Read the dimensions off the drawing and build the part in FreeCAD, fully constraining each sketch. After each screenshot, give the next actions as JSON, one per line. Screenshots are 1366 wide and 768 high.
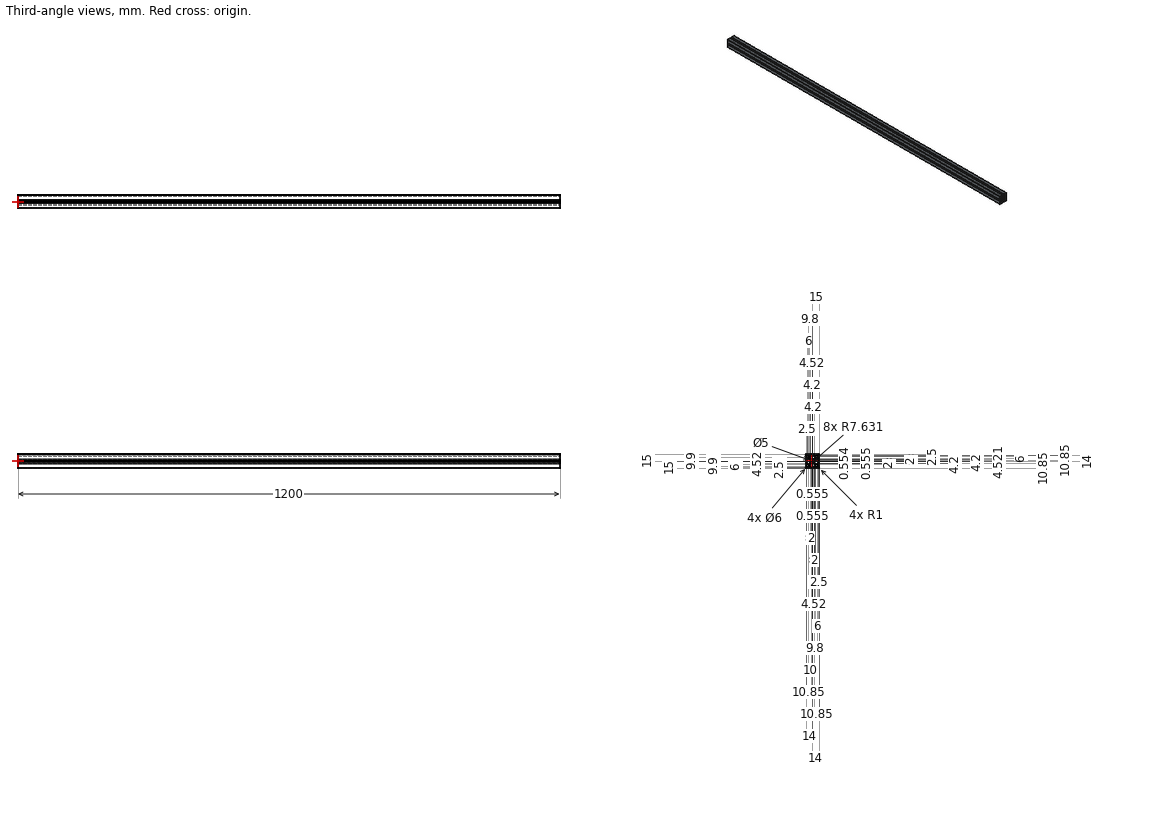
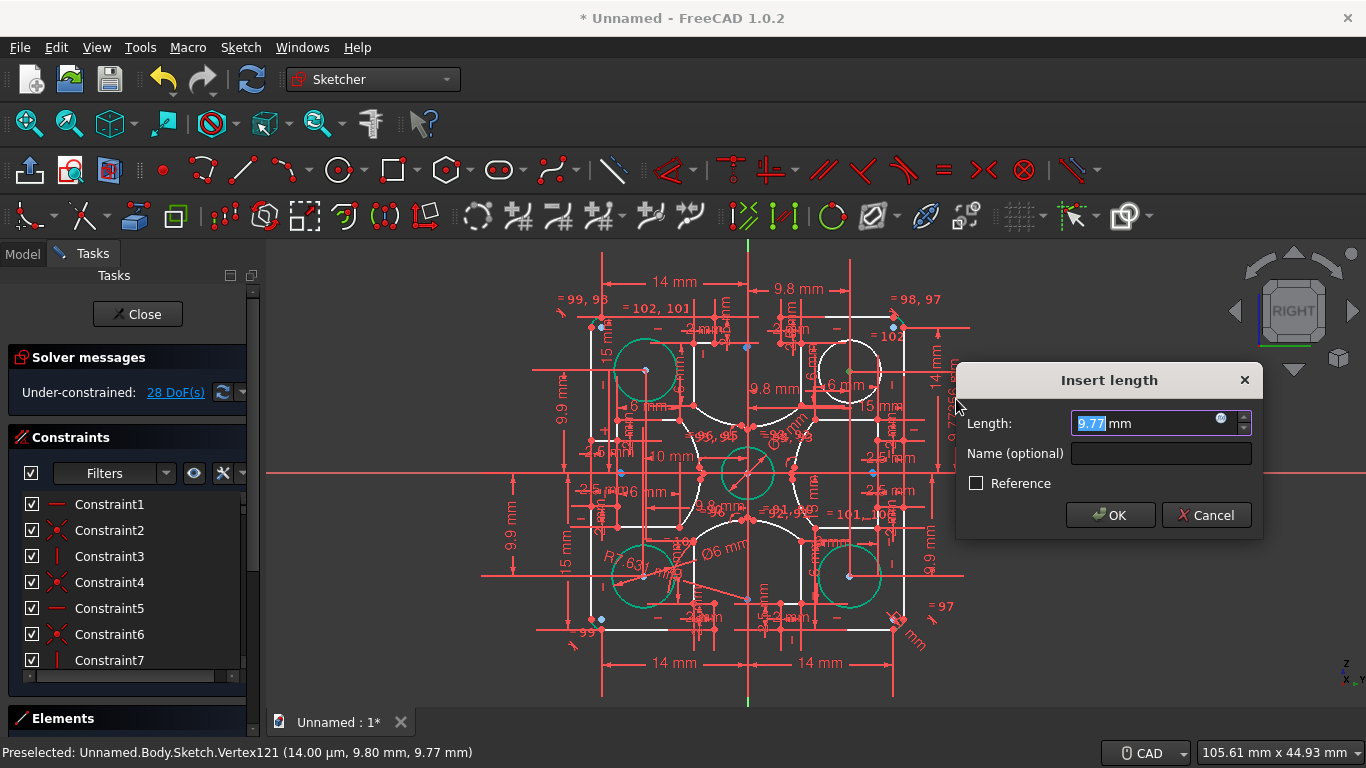
{"action": "type", "text": "9.9"}
{"action": "key", "text": "Return"}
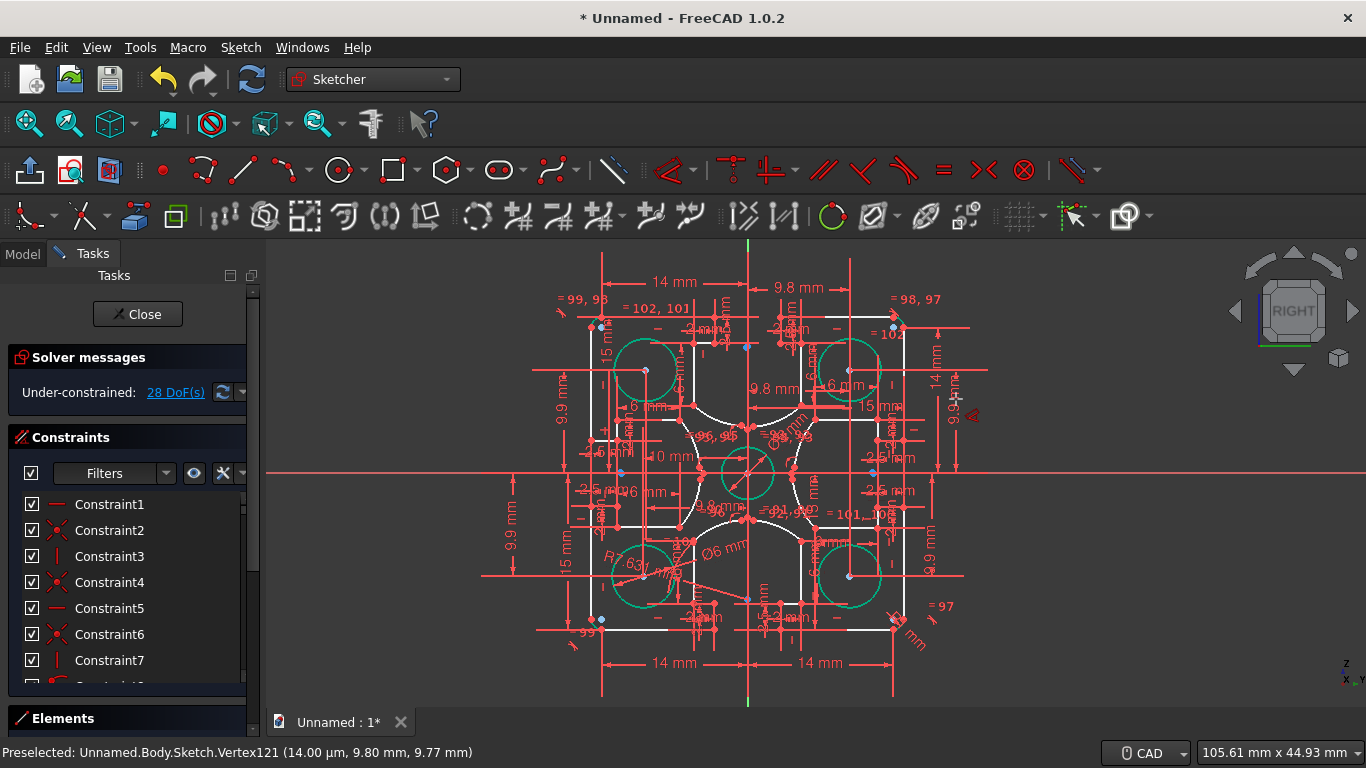
{"action": "scroll", "coordinate": [748, 517], "scroll_direction": "up", "scroll_amount": 4}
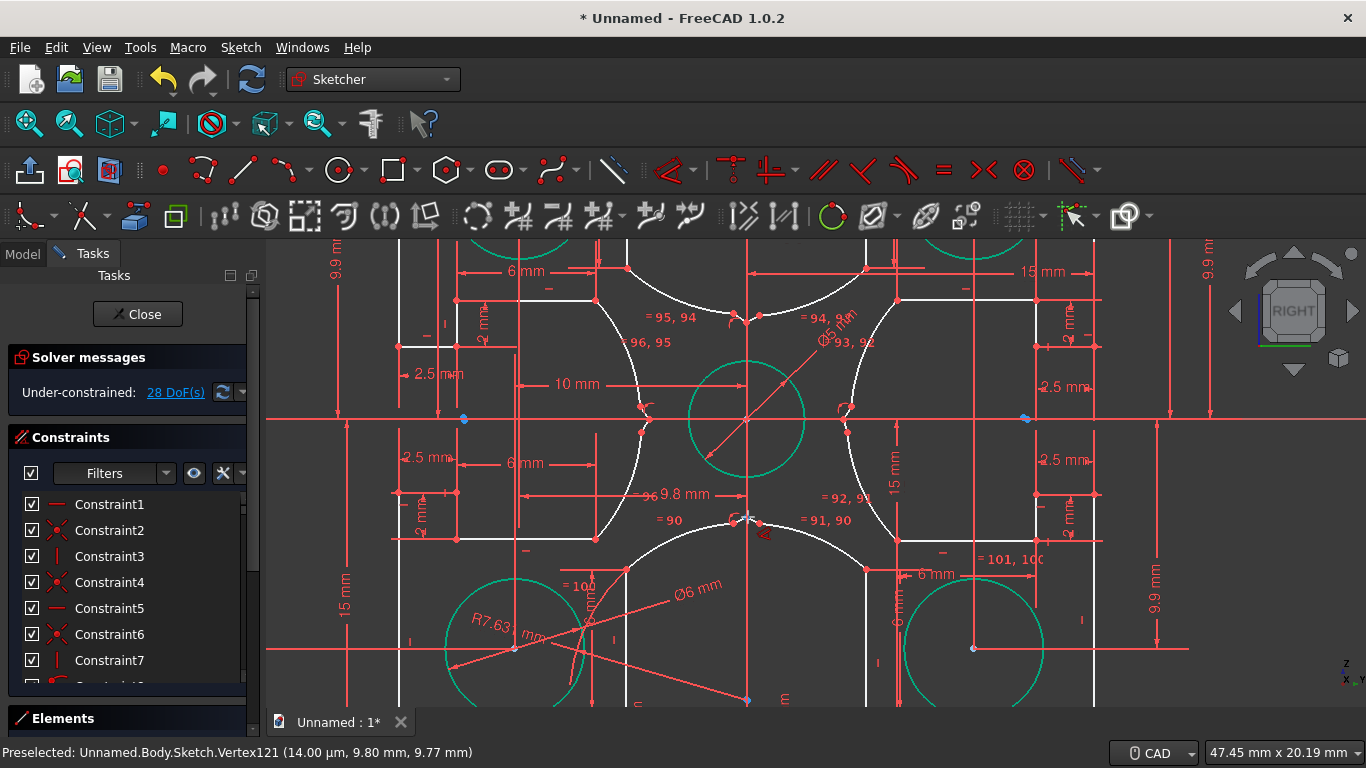
{"action": "left_click", "coordinate": [747, 517]}
{"action": "left_click", "coordinate": [781, 446]}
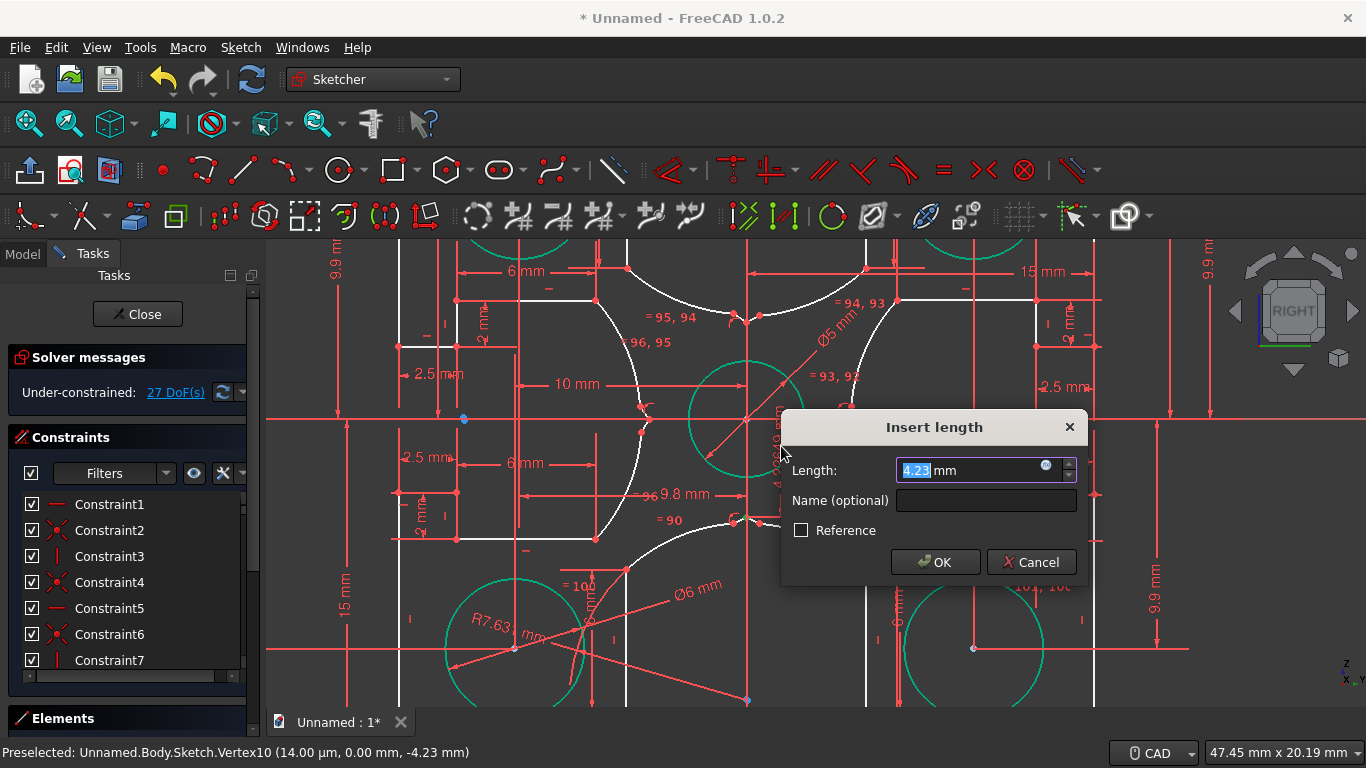
{"action": "type", "text": "4.2"}
{"action": "key", "text": "Return"}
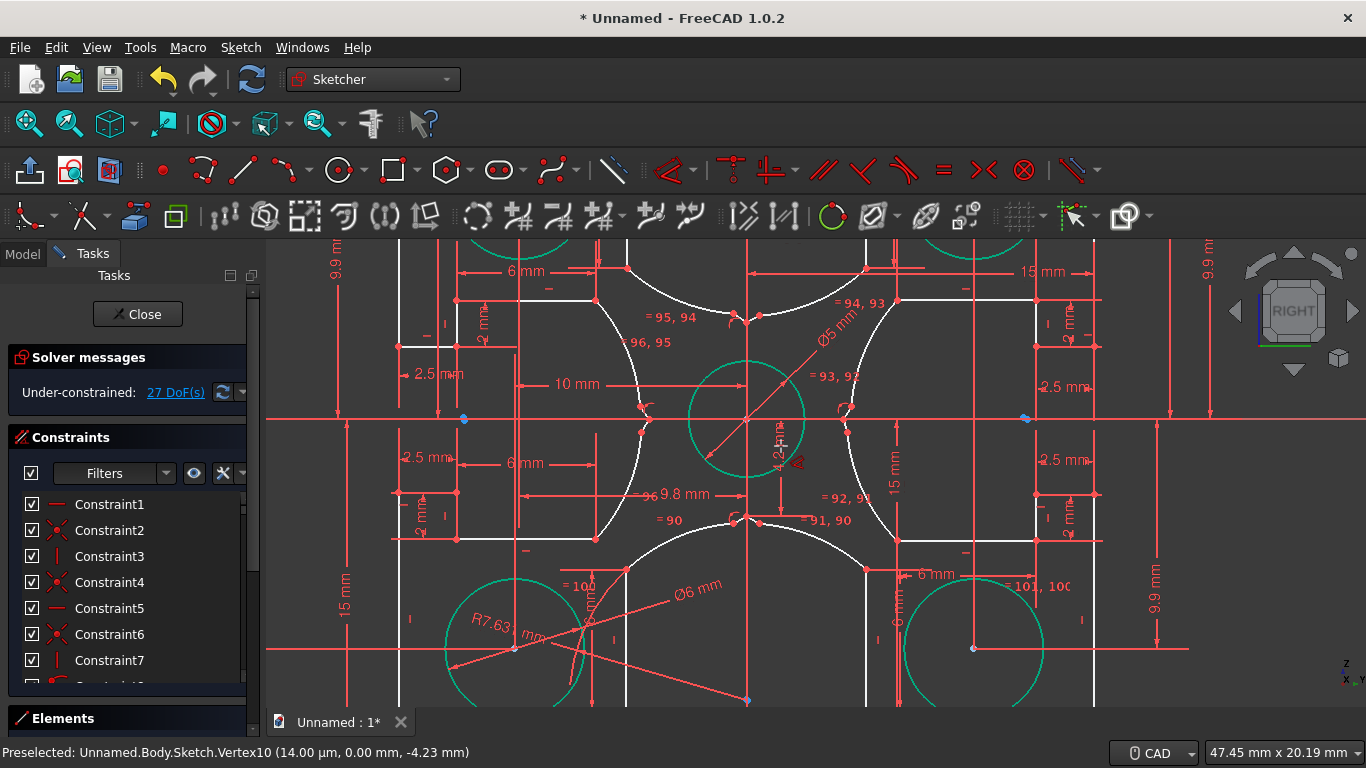
{"action": "left_click", "coordinate": [844, 419]}
{"action": "left_click", "coordinate": [773, 385]}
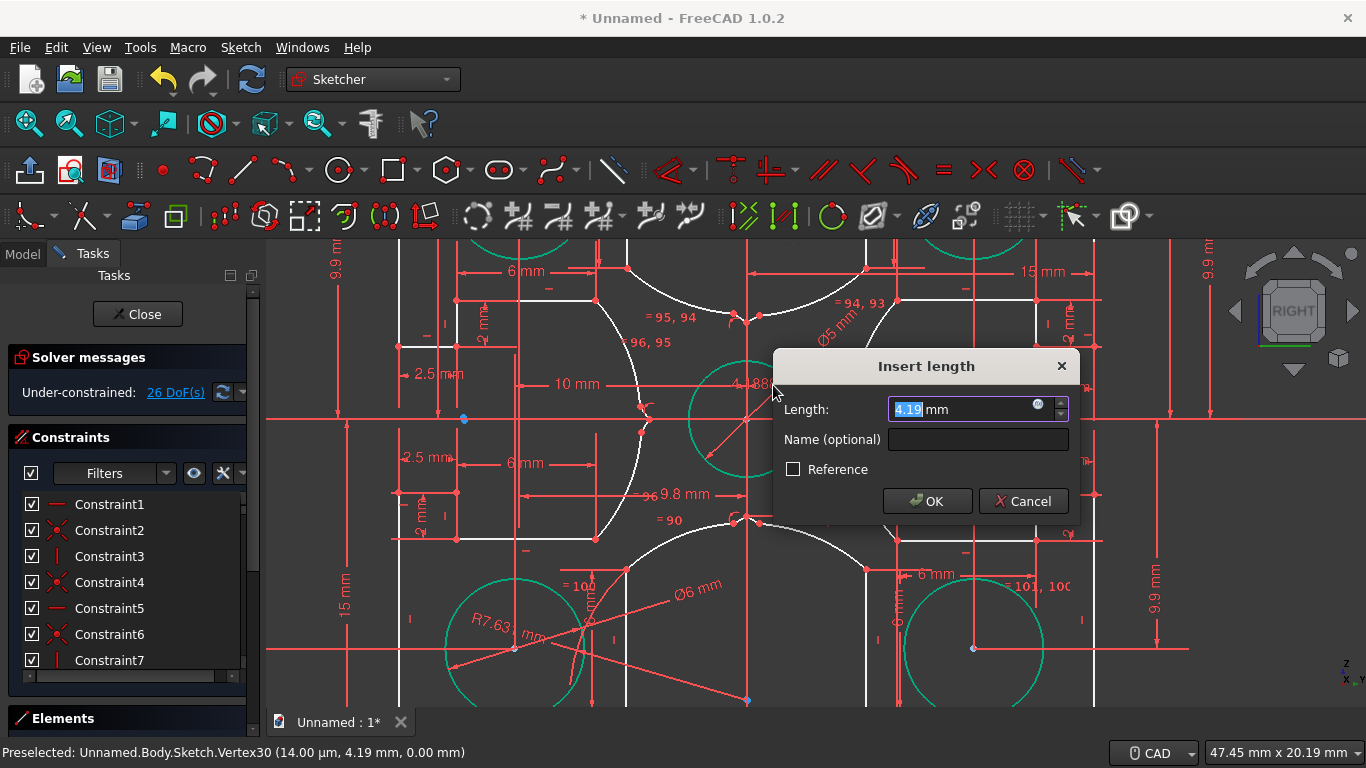
{"action": "type", "text": "4.2"}
{"action": "key", "text": "Return"}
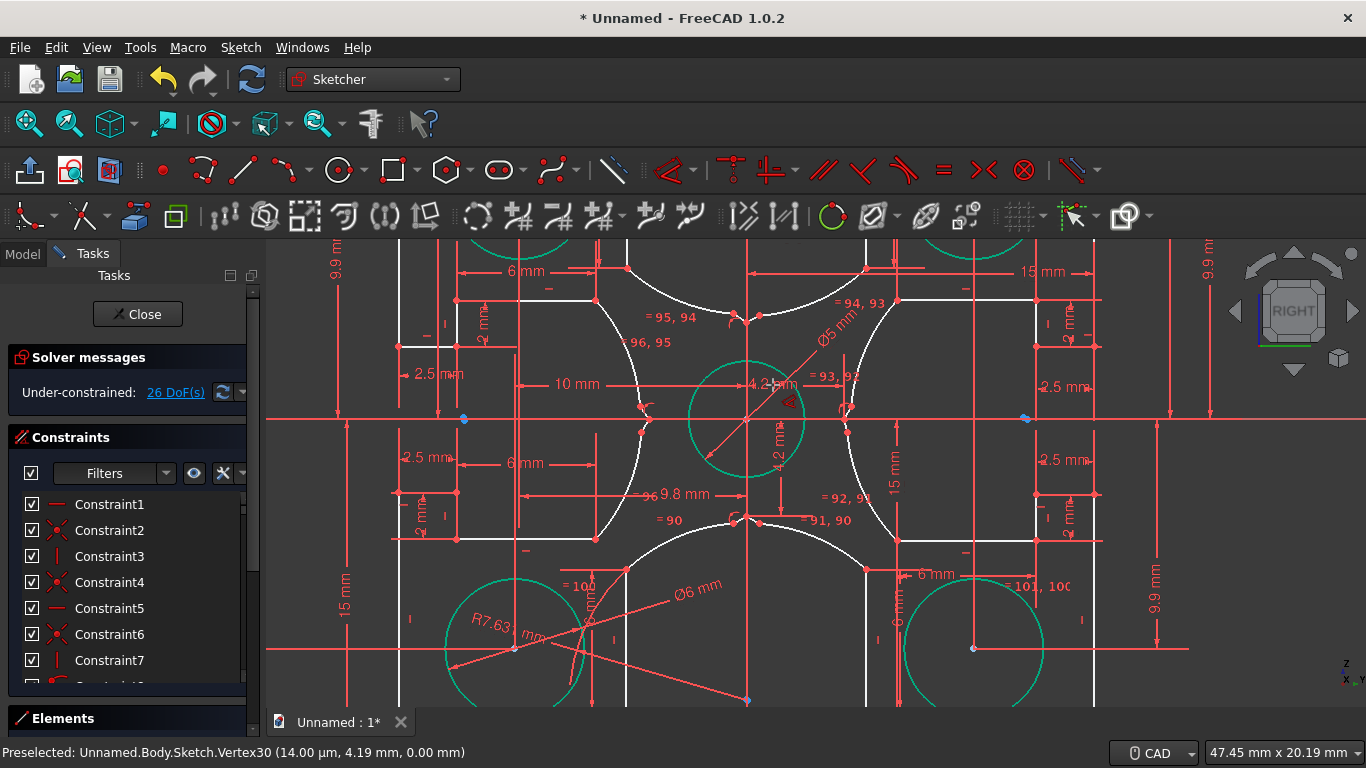
{"action": "left_click", "coordinate": [747, 322]}
{"action": "left_click", "coordinate": [781, 348]}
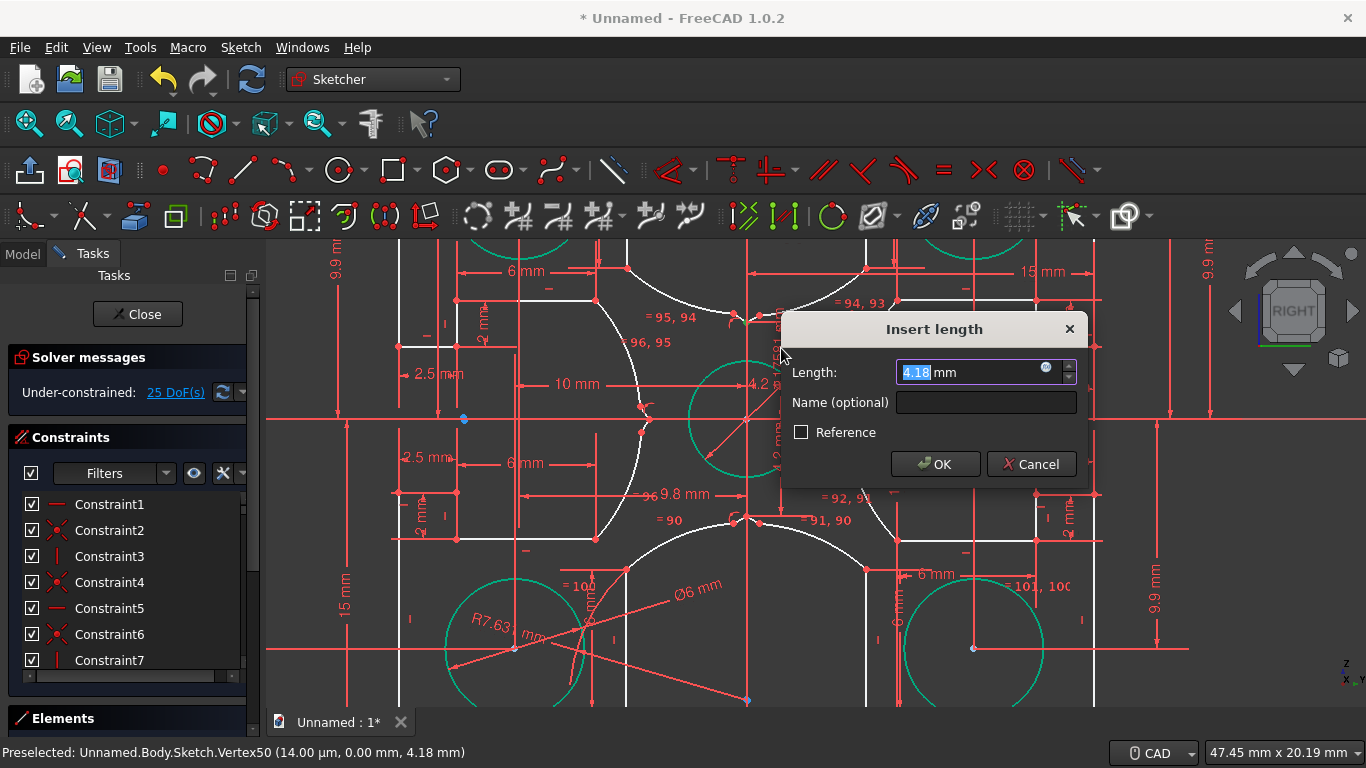
{"action": "type", "text": "4.2"}
{"action": "key", "text": "Return"}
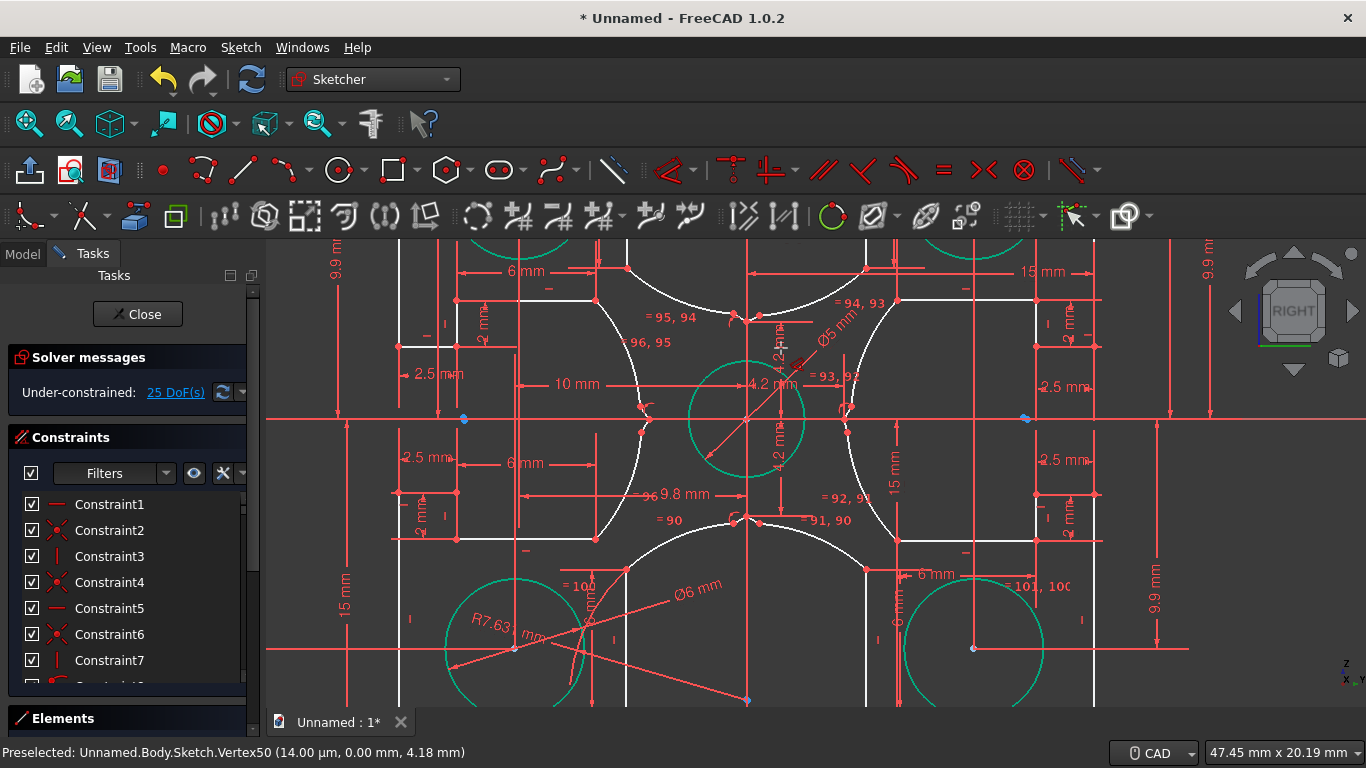
{"action": "left_click", "coordinate": [649, 419]}
{"action": "left_click", "coordinate": [675, 453]}